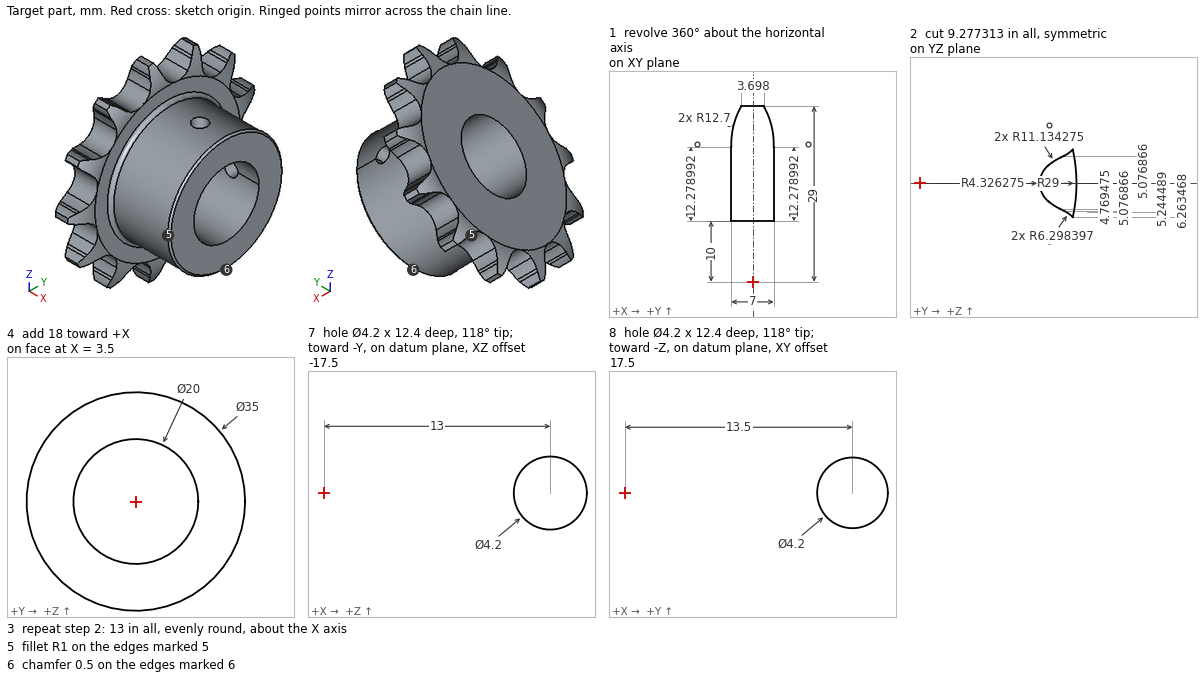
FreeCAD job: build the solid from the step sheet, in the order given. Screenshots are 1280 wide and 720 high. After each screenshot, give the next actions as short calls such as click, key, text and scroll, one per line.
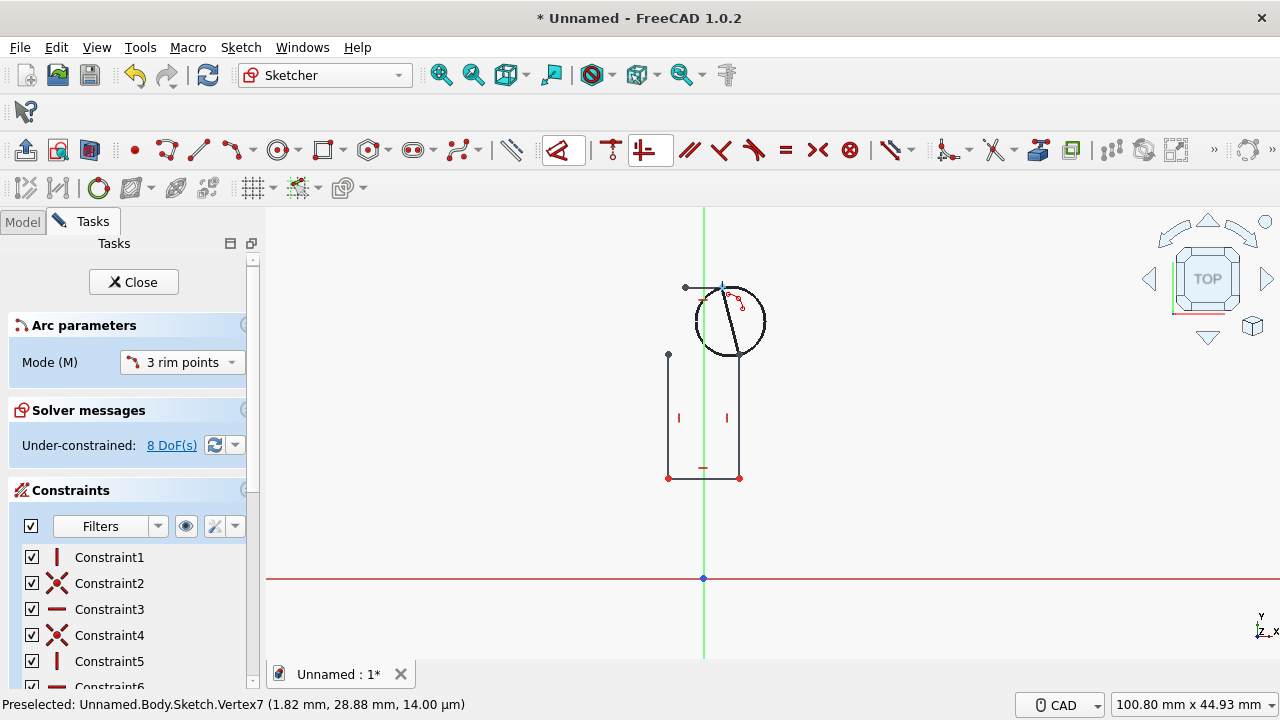
scroll(735, 319, up, 6)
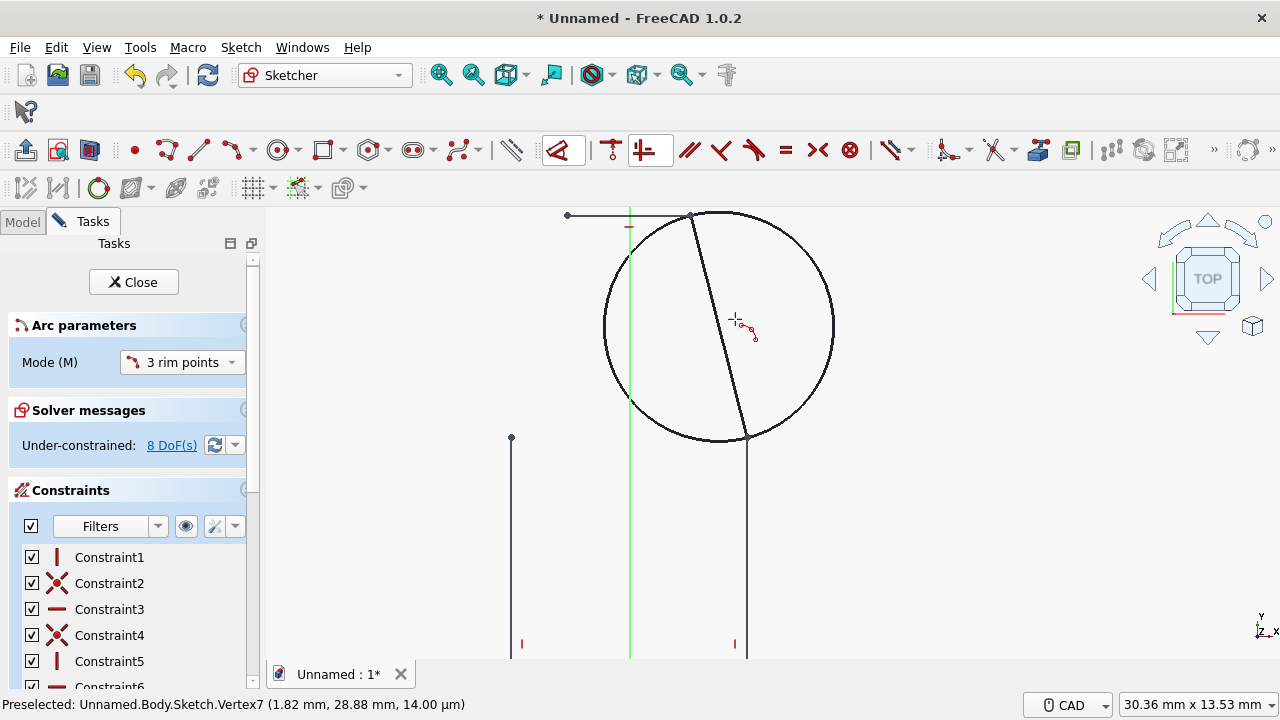
click(735, 320)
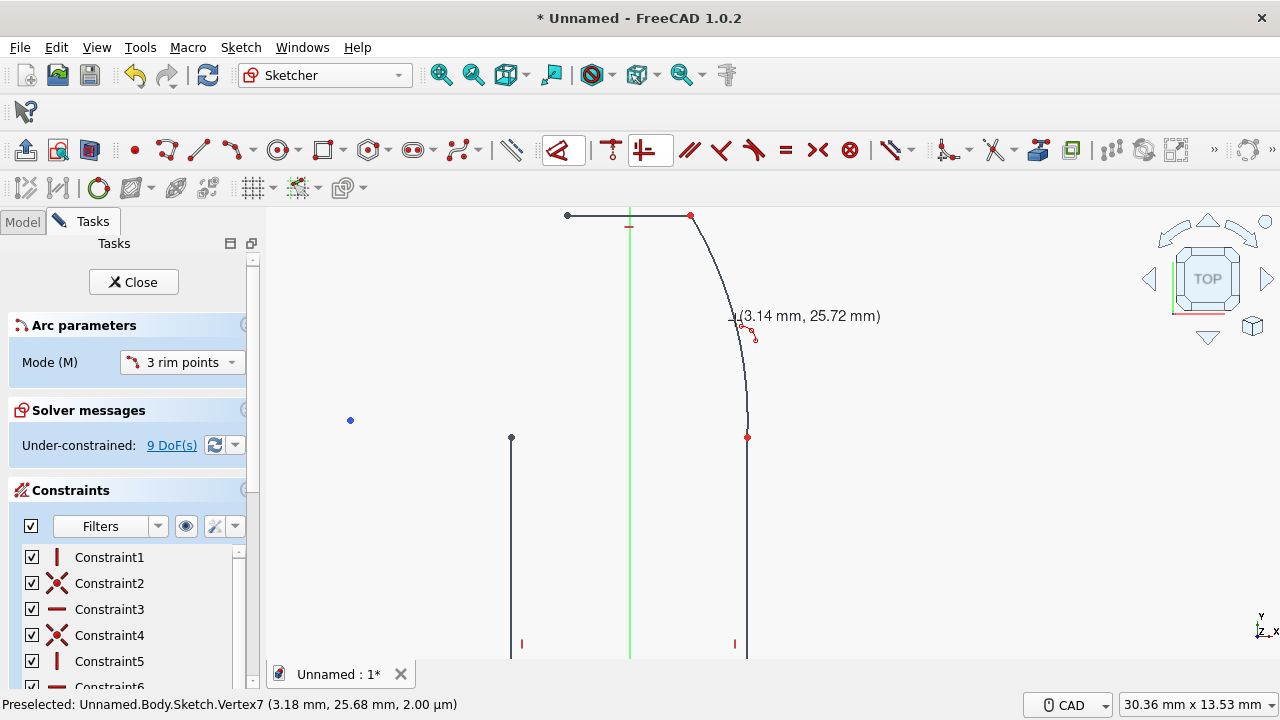
scroll(737, 320, down, 6)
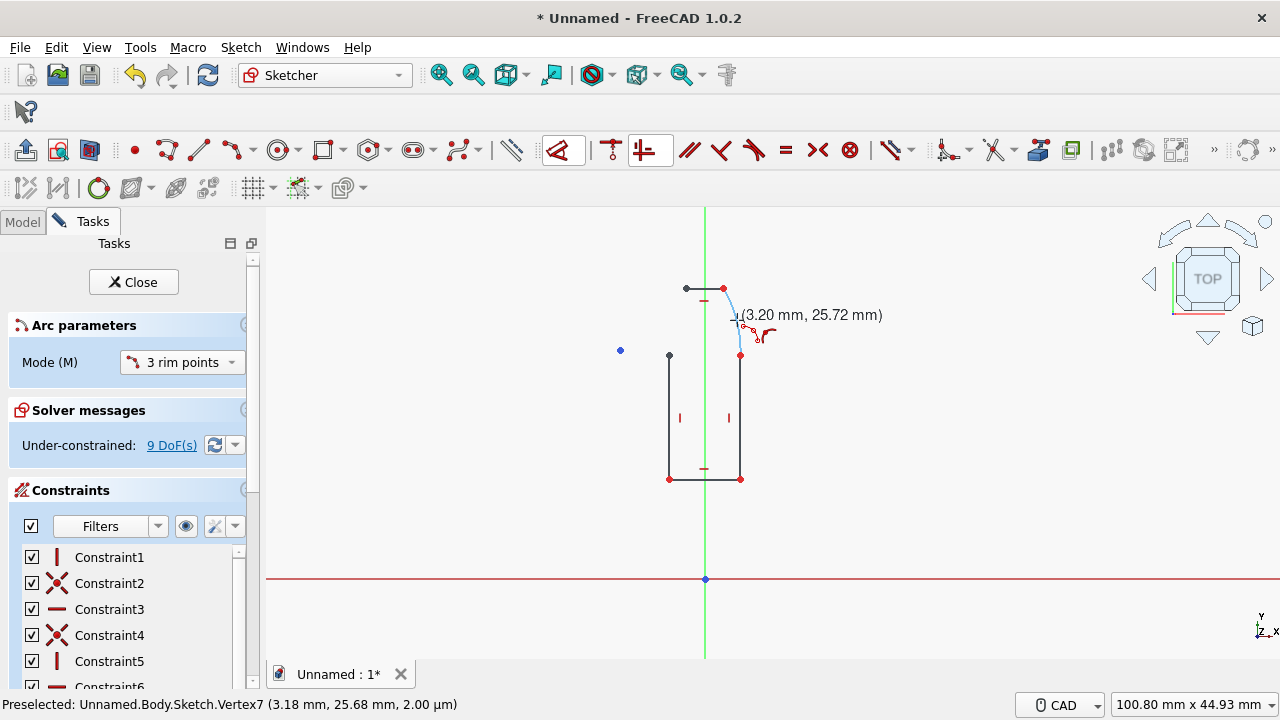
click(686, 289)
click(669, 356)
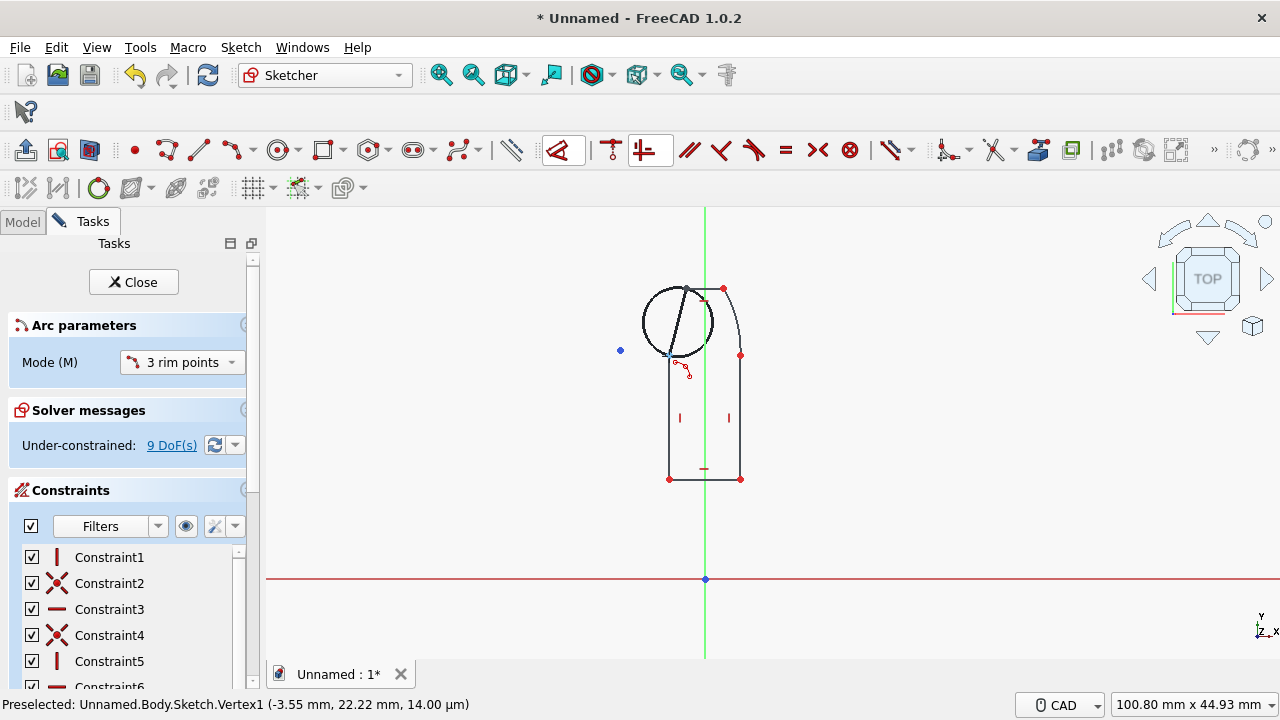
scroll(673, 320, up, 6)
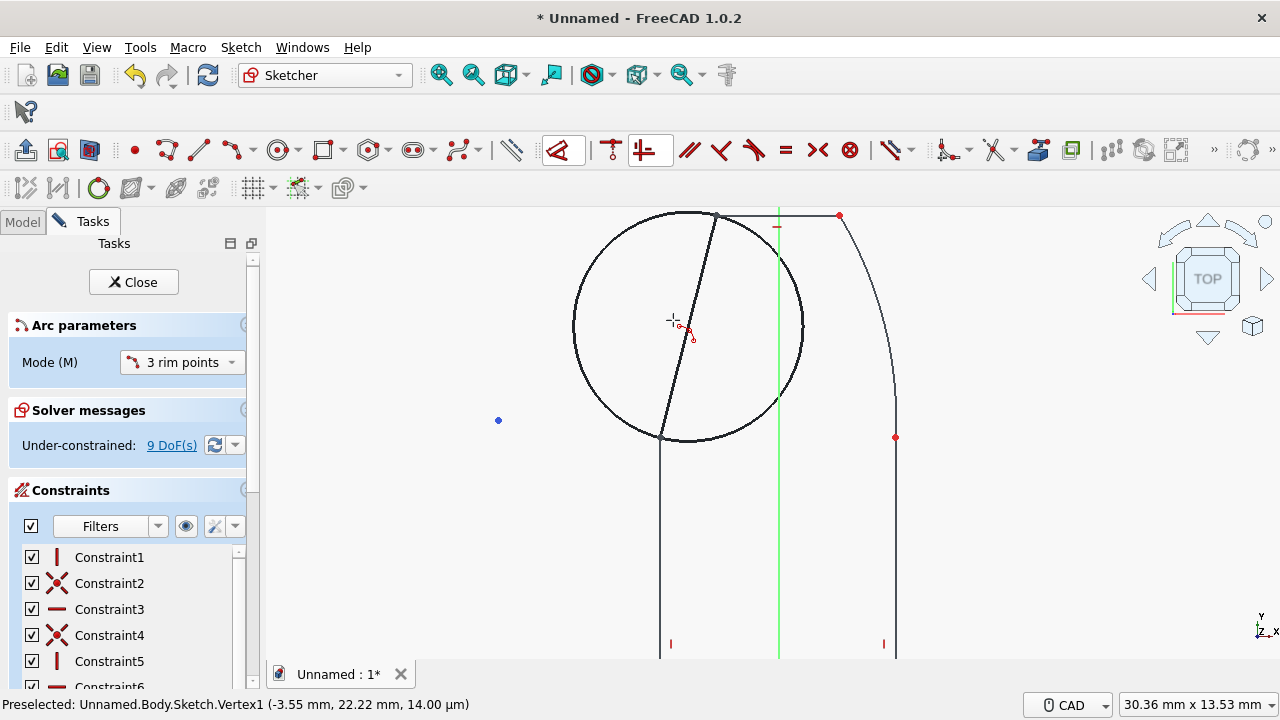
click(674, 320)
key(Escape)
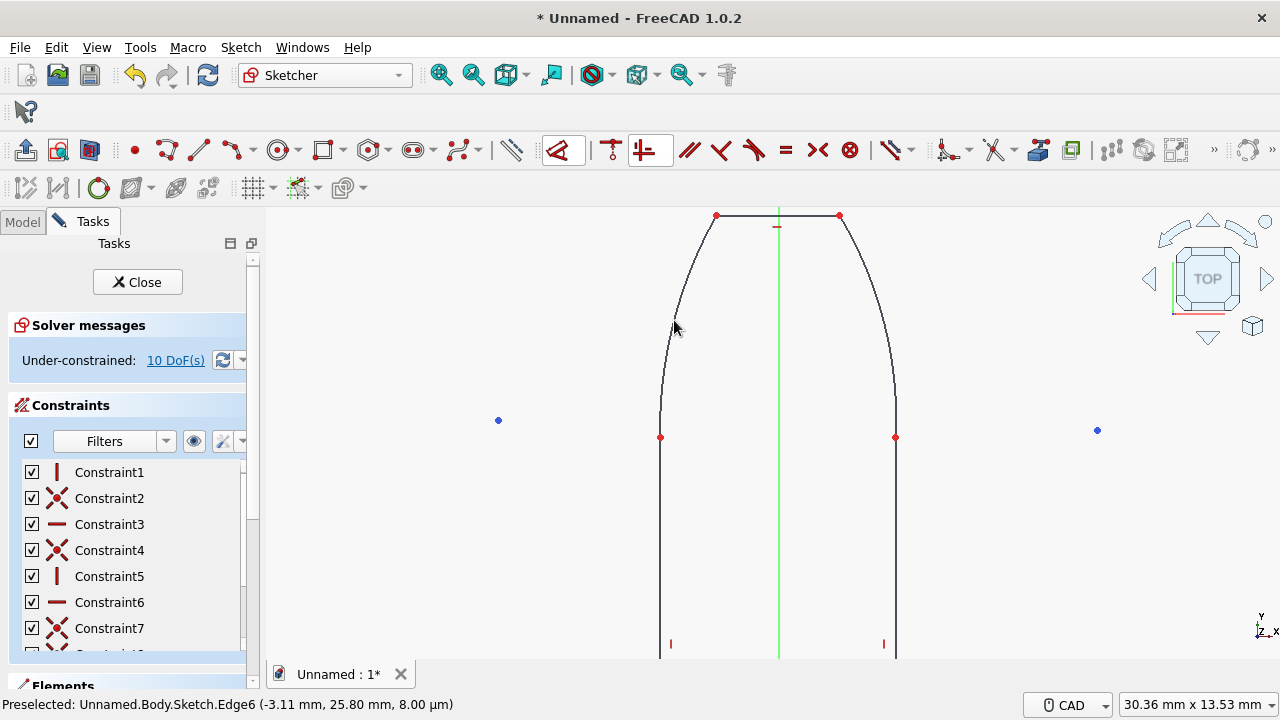
click(893, 368)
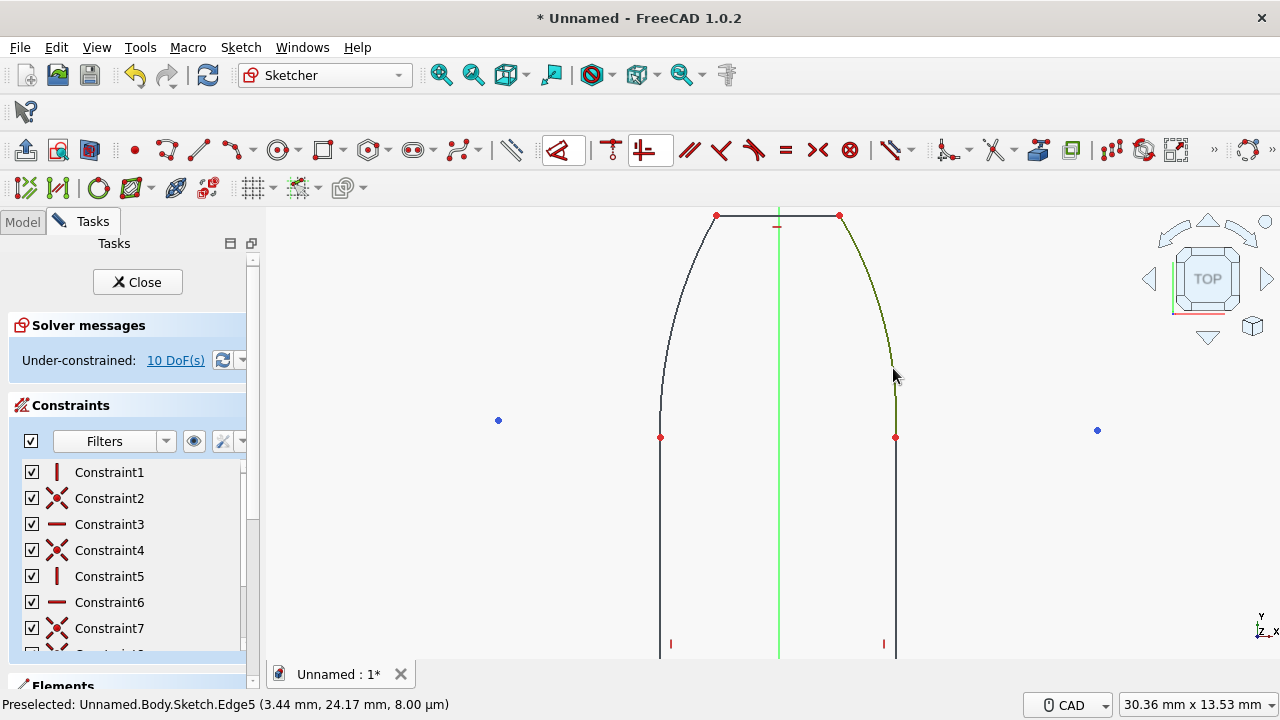
click(687, 279)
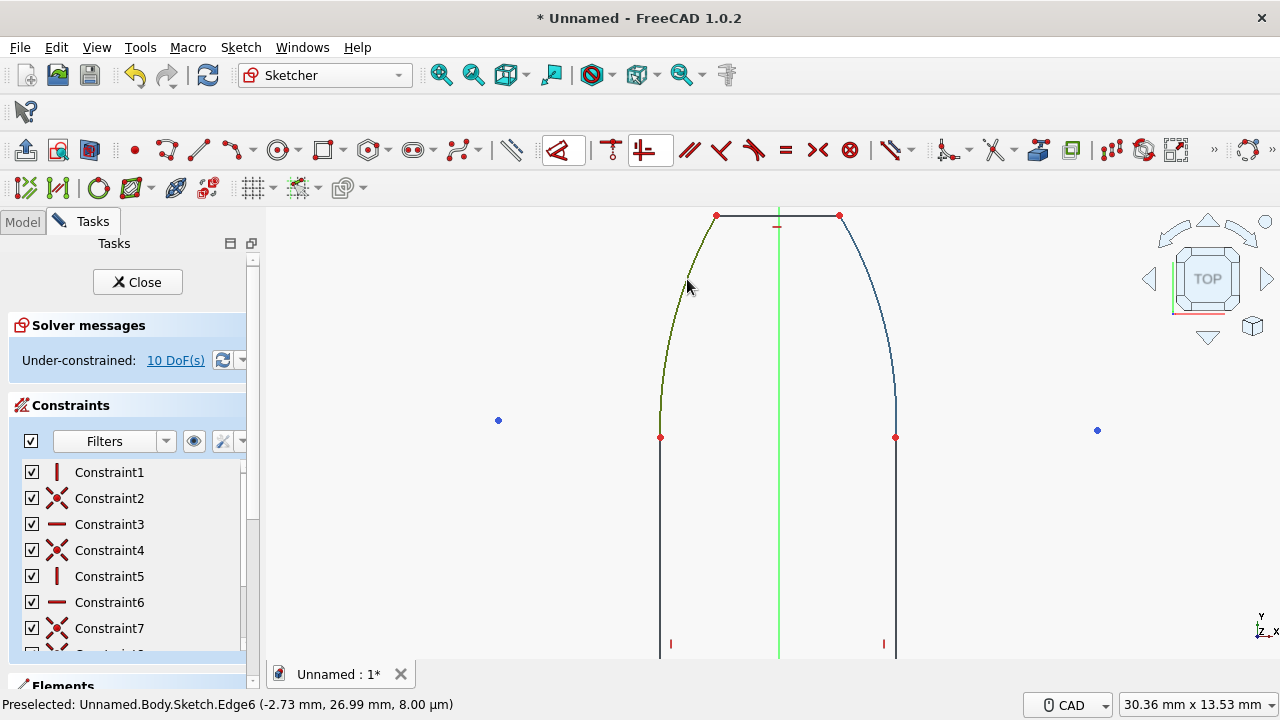
key(e)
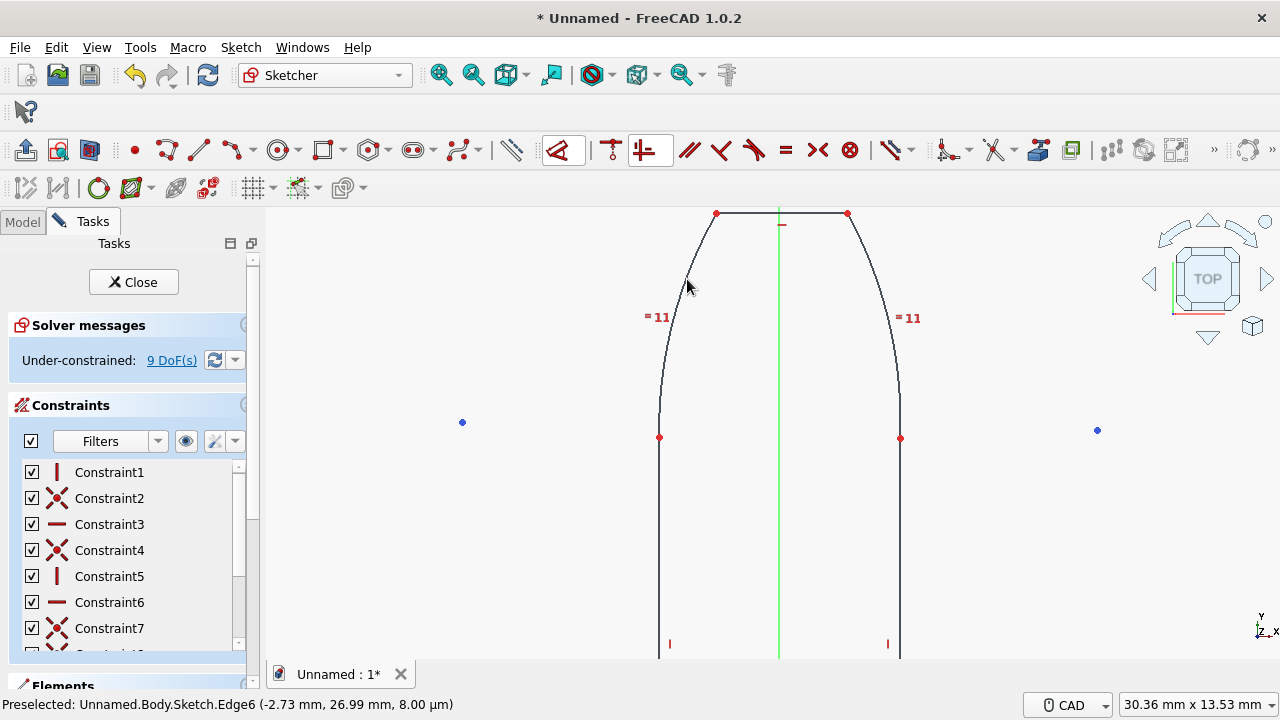
click(462, 422)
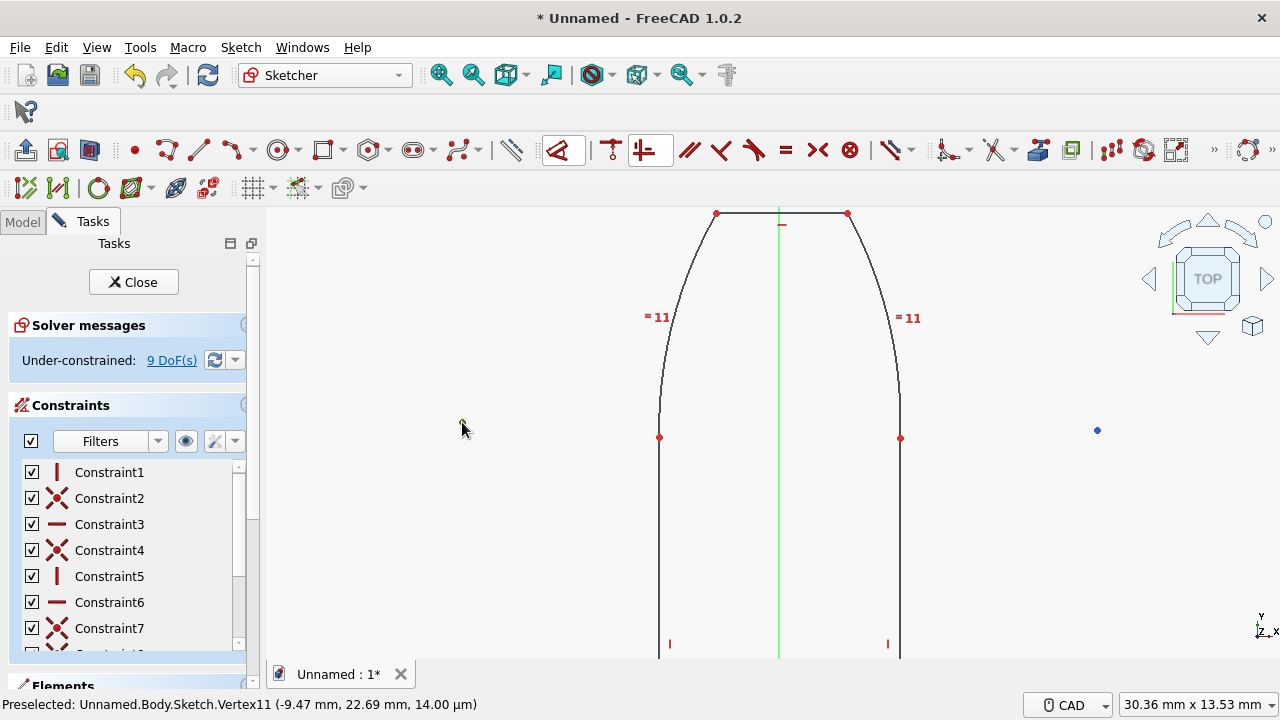
click(1097, 430)